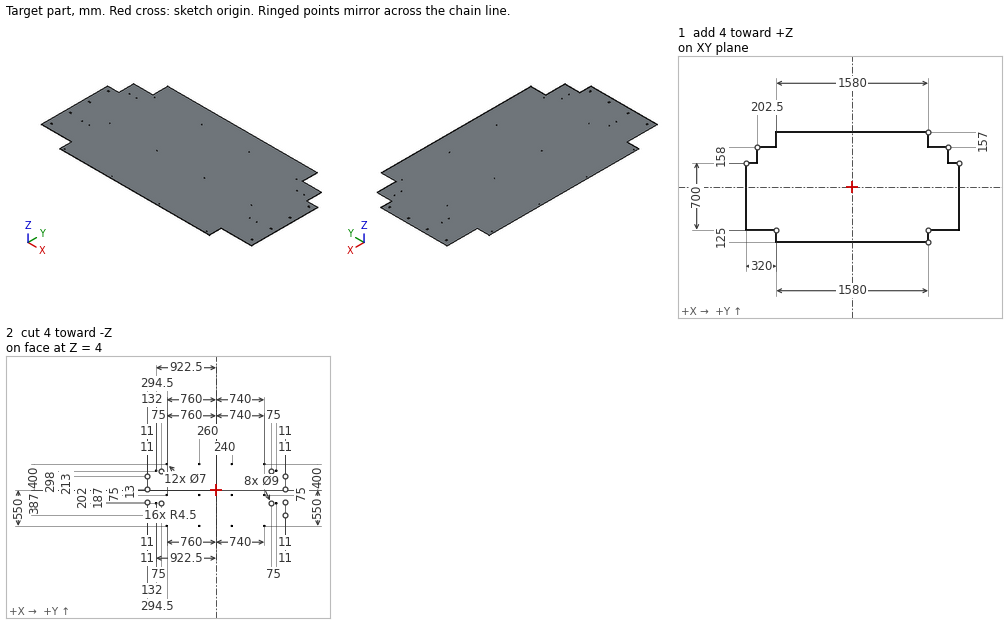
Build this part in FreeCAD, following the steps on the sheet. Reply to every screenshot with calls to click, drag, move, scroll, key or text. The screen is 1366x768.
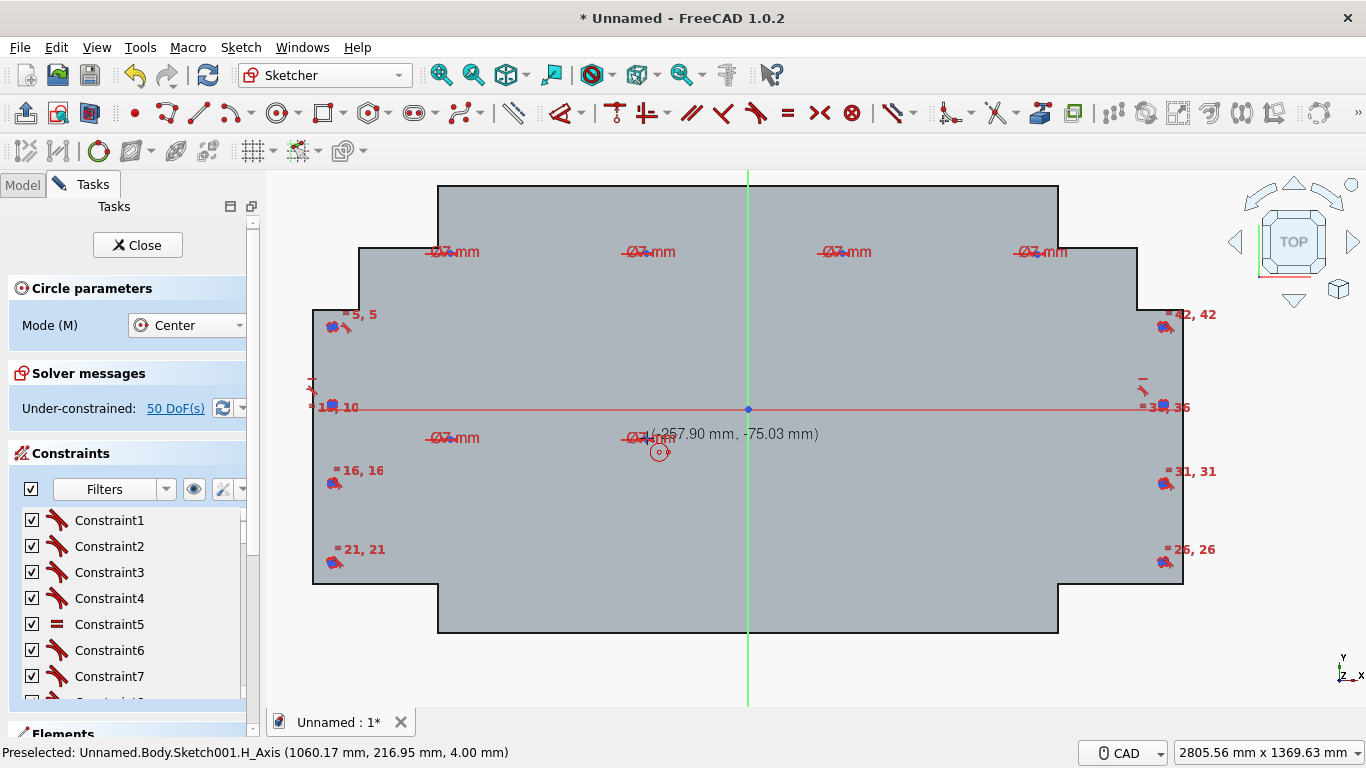
scroll(842, 439, up, 15)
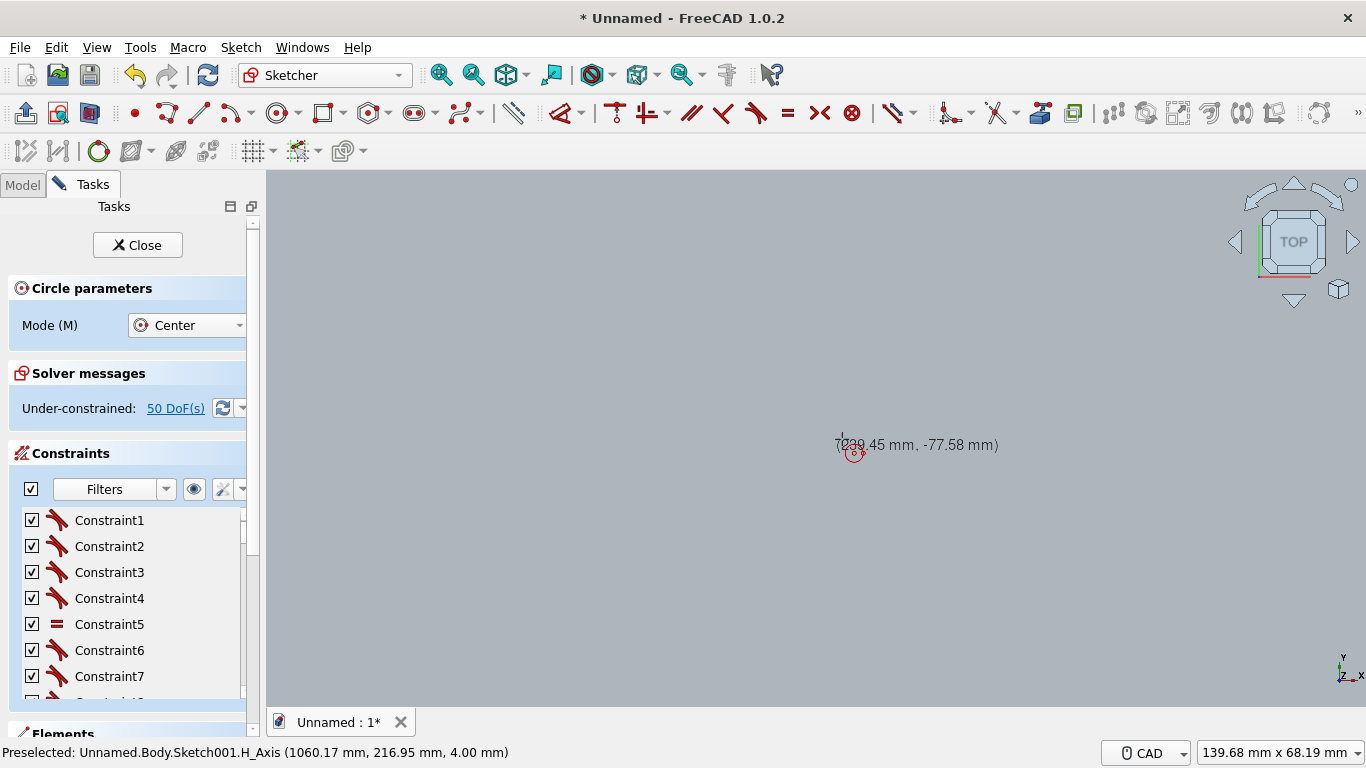
scroll(842, 439, down, 15)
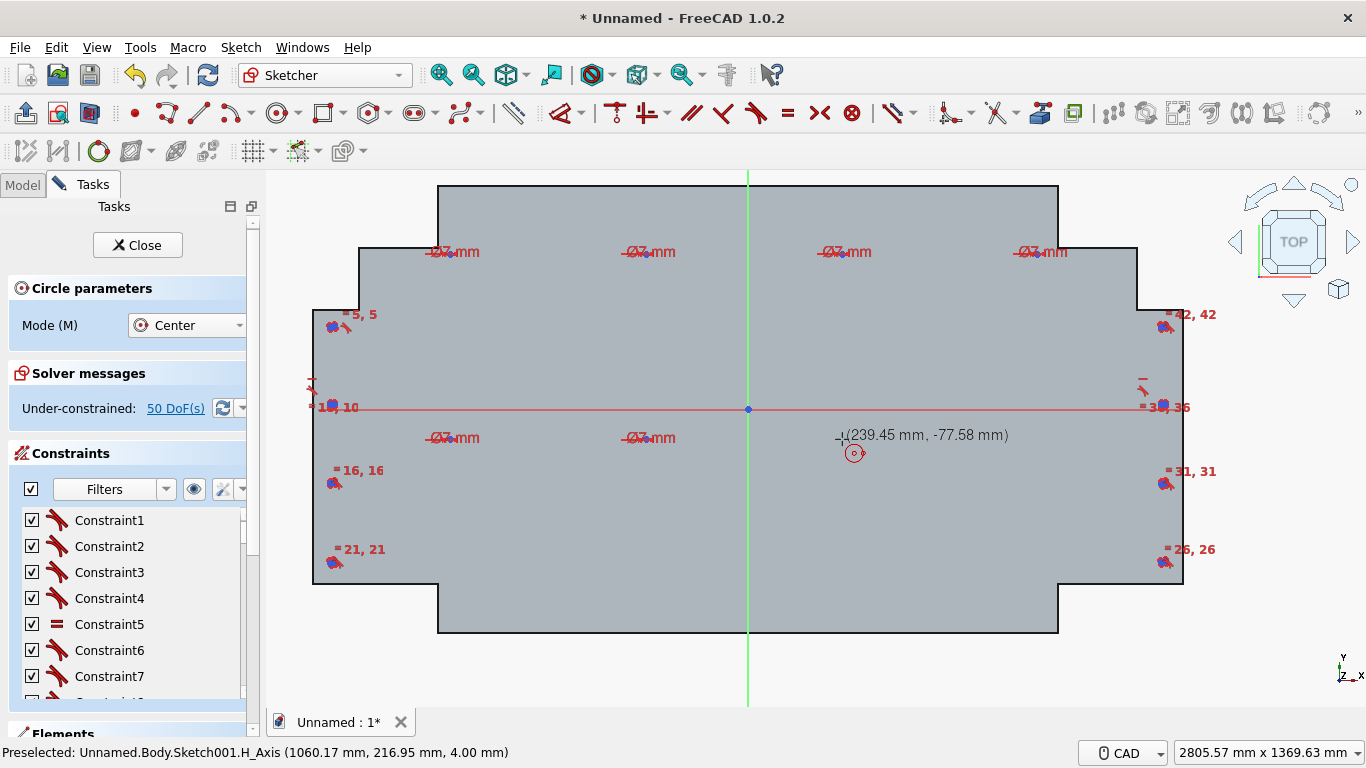
click(842, 439)
move(843, 438)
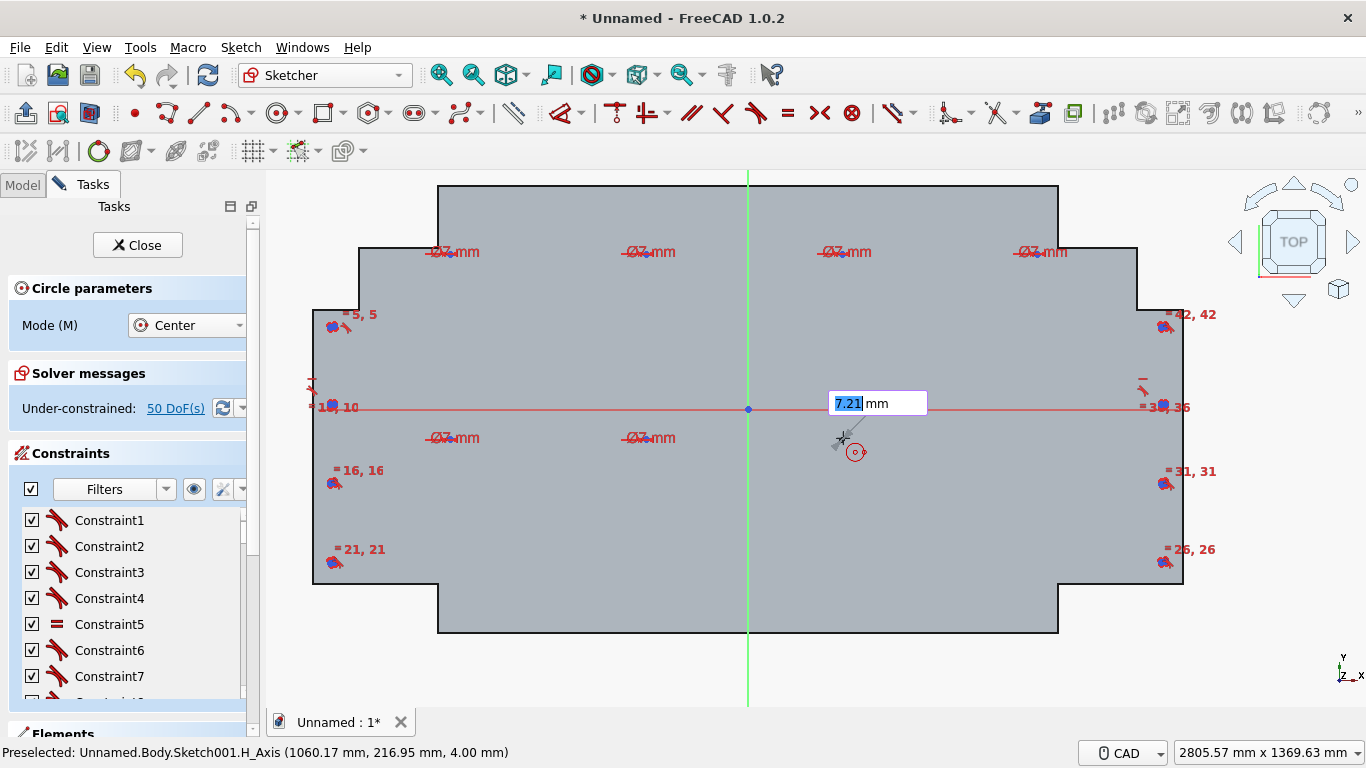
text(7)
key(Return)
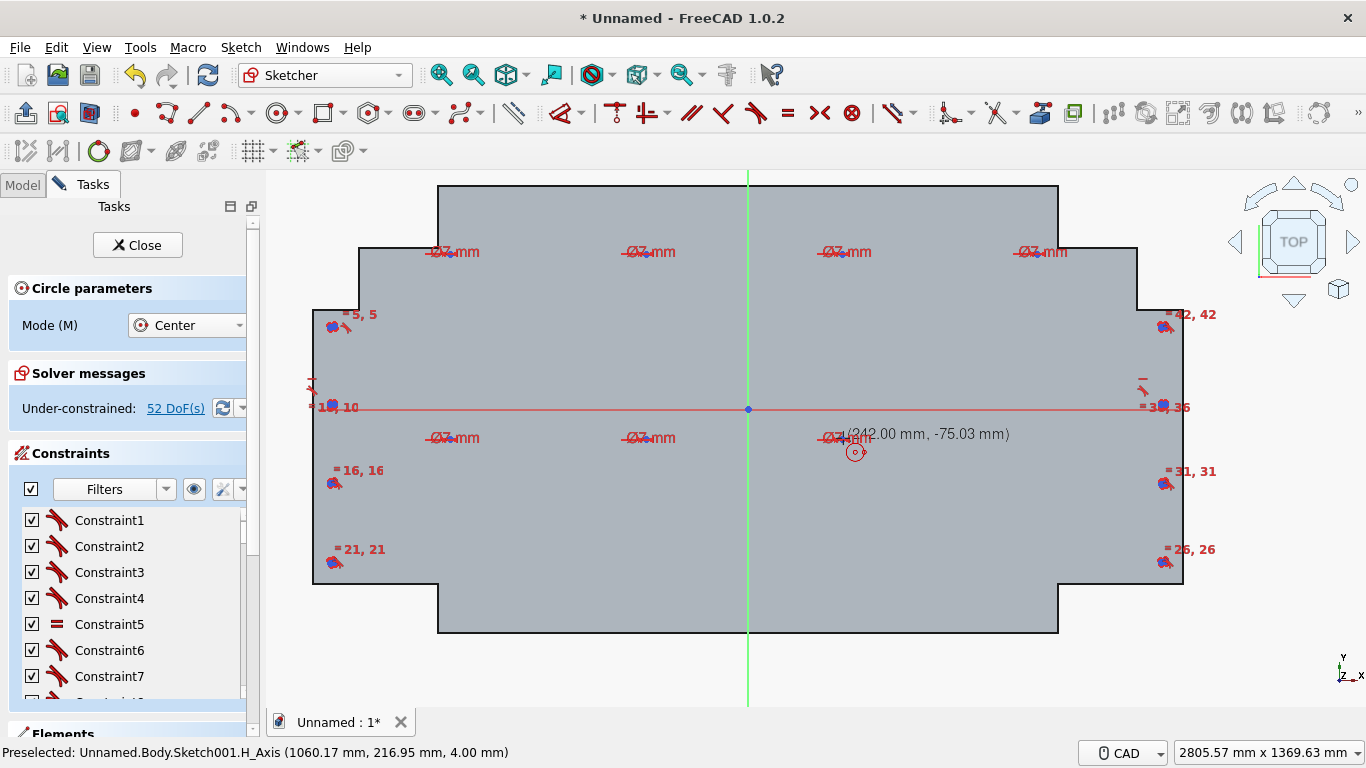
scroll(1038, 439, up, 15)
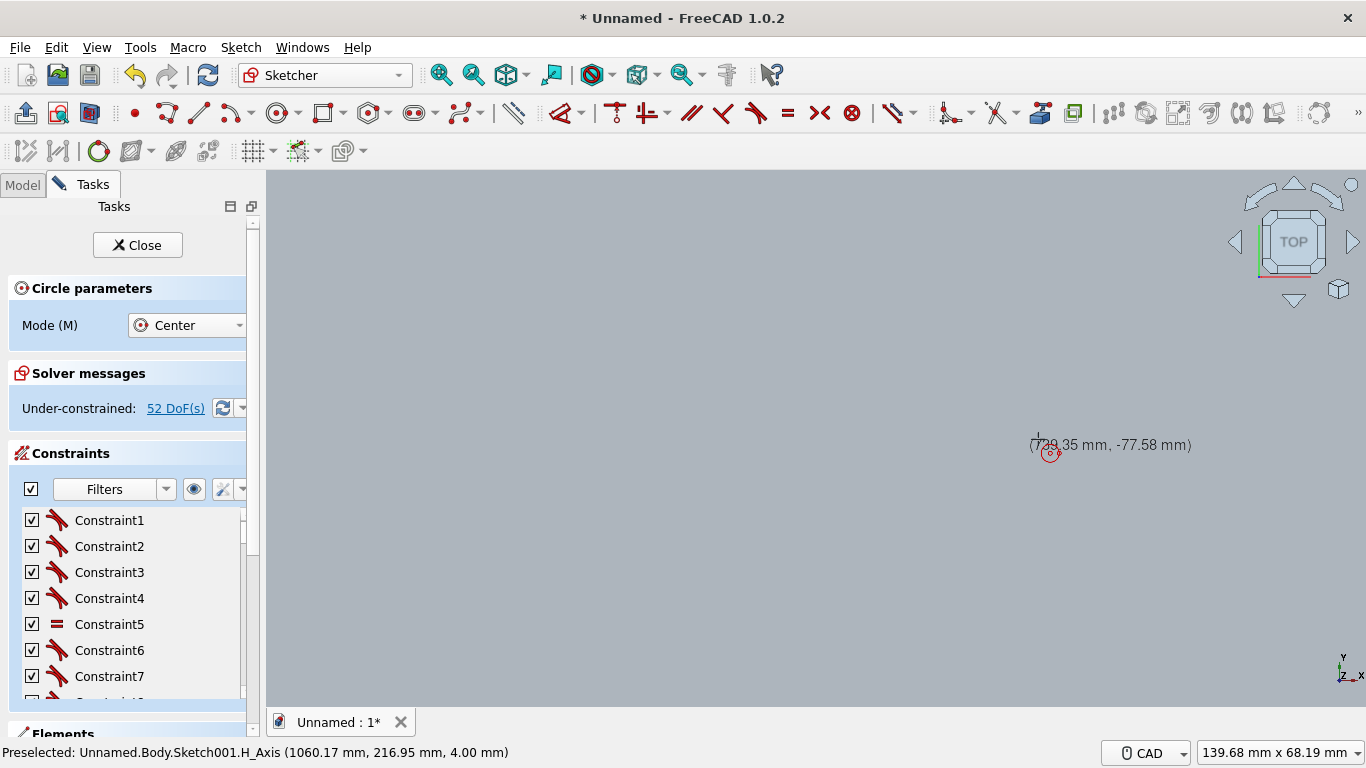
scroll(1038, 439, down, 15)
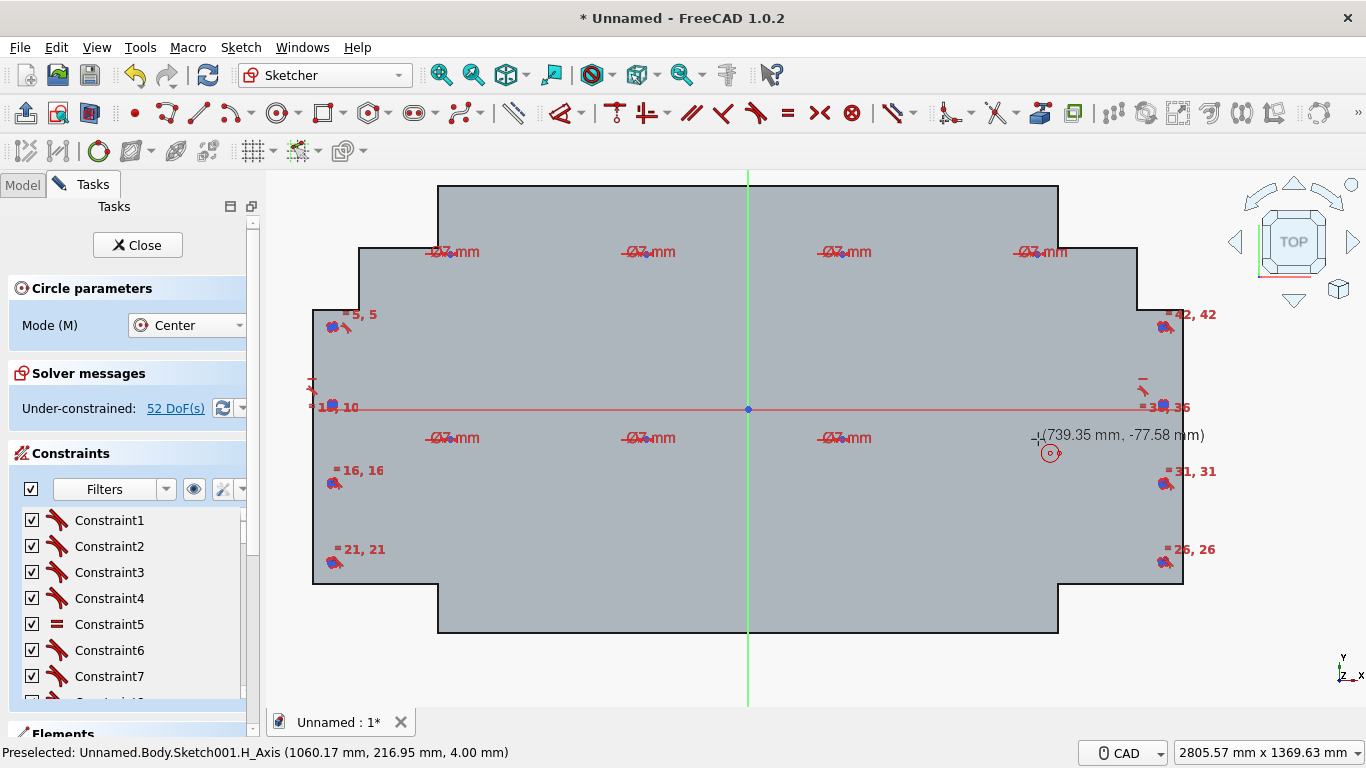
click(1038, 439)
move(1039, 438)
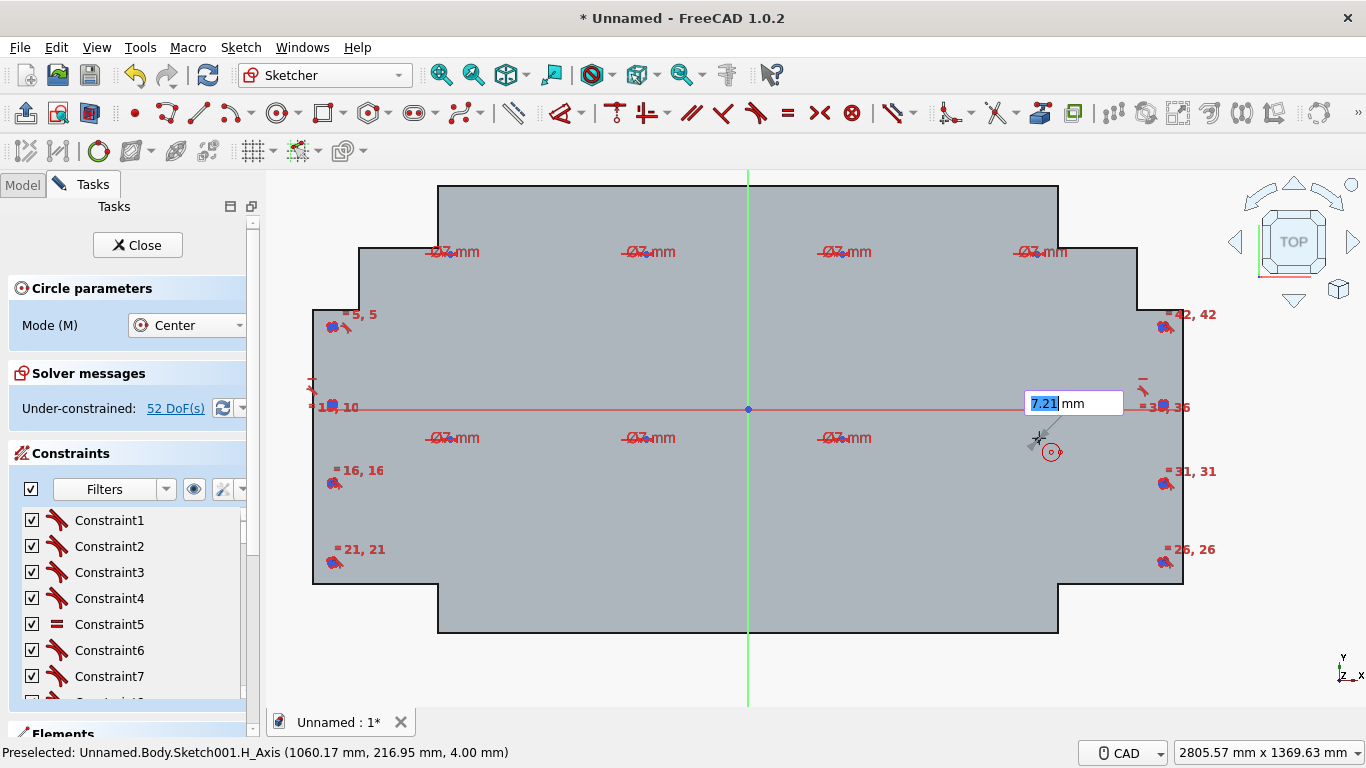
text(7)
key(Return)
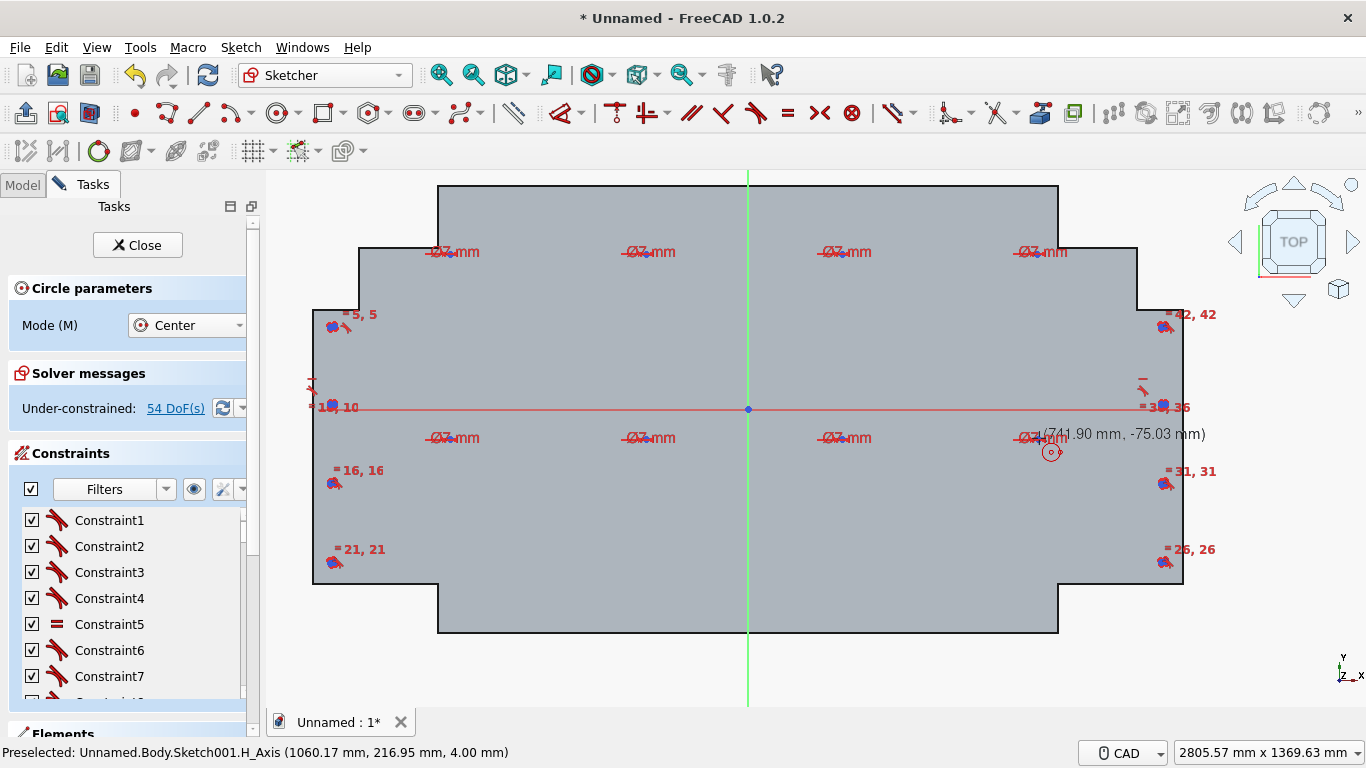
scroll(450, 625, up, 15)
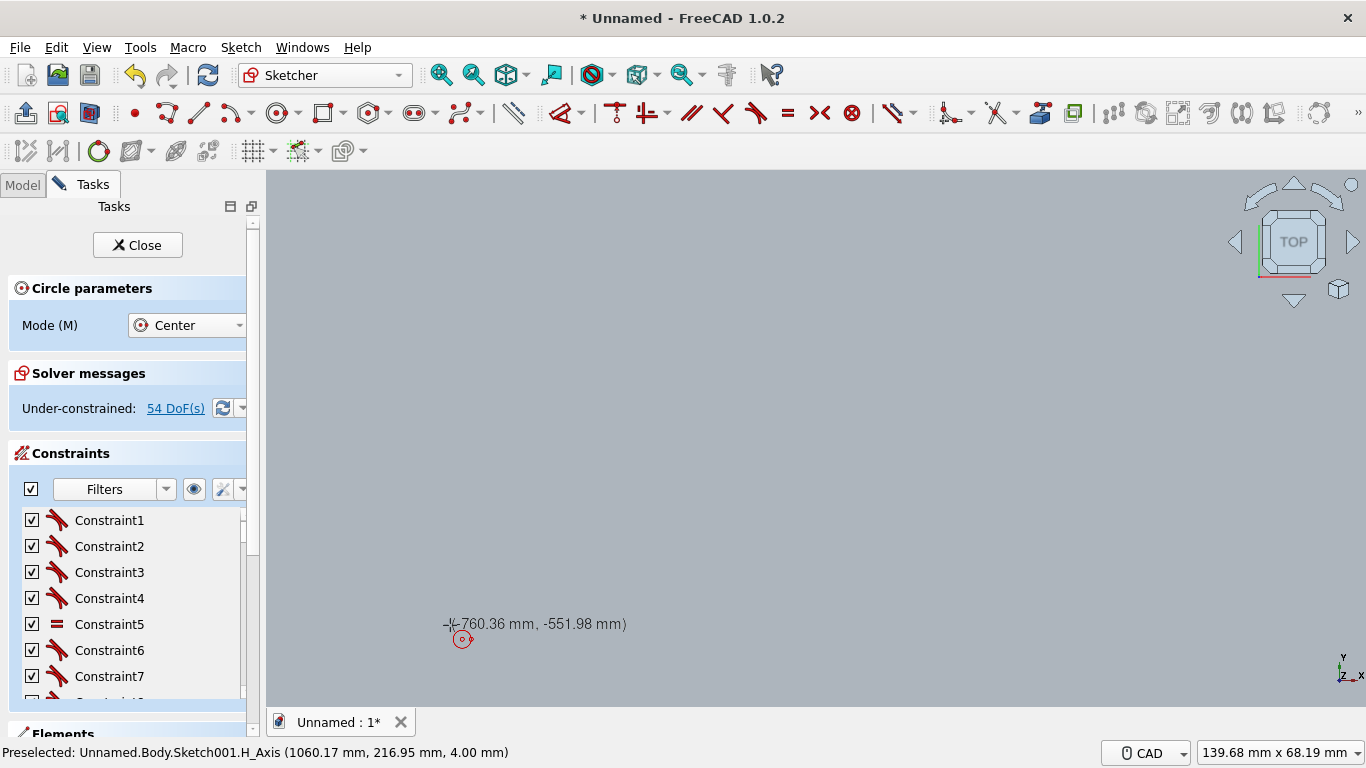
scroll(450, 625, down, 15)